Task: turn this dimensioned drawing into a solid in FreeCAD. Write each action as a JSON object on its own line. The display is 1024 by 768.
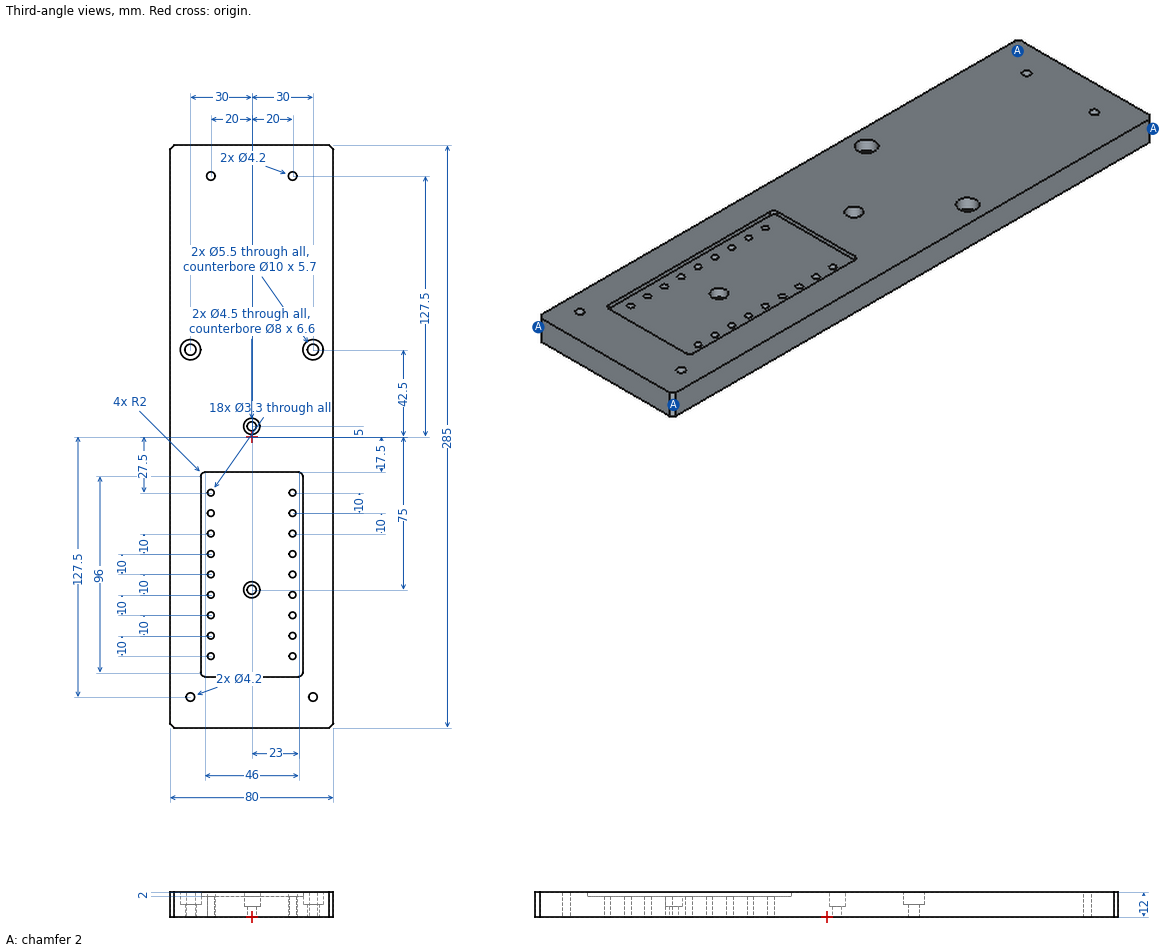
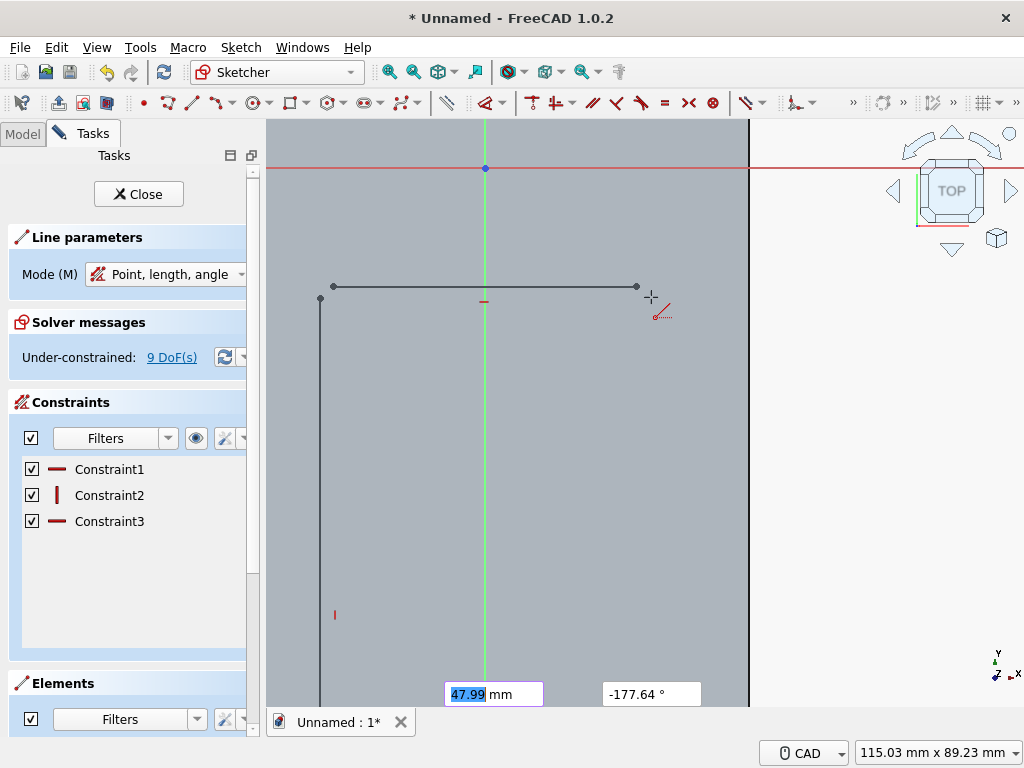
{"action": "left_click", "coordinate": [650, 297]}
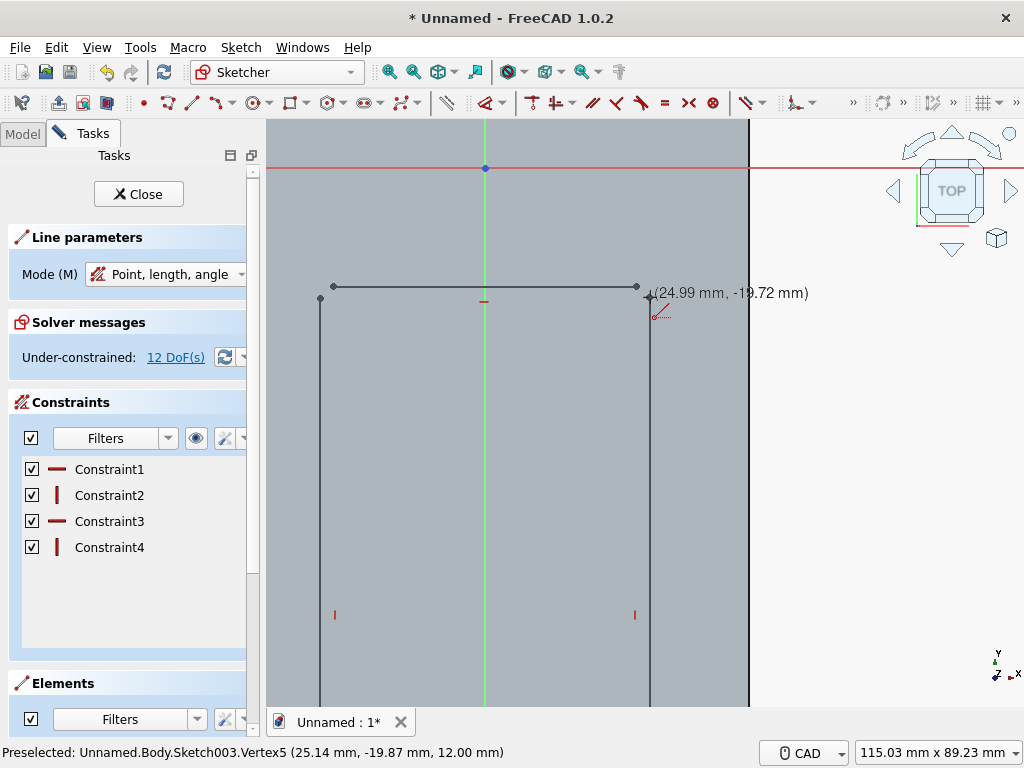
{"action": "key", "text": "g 3 a"}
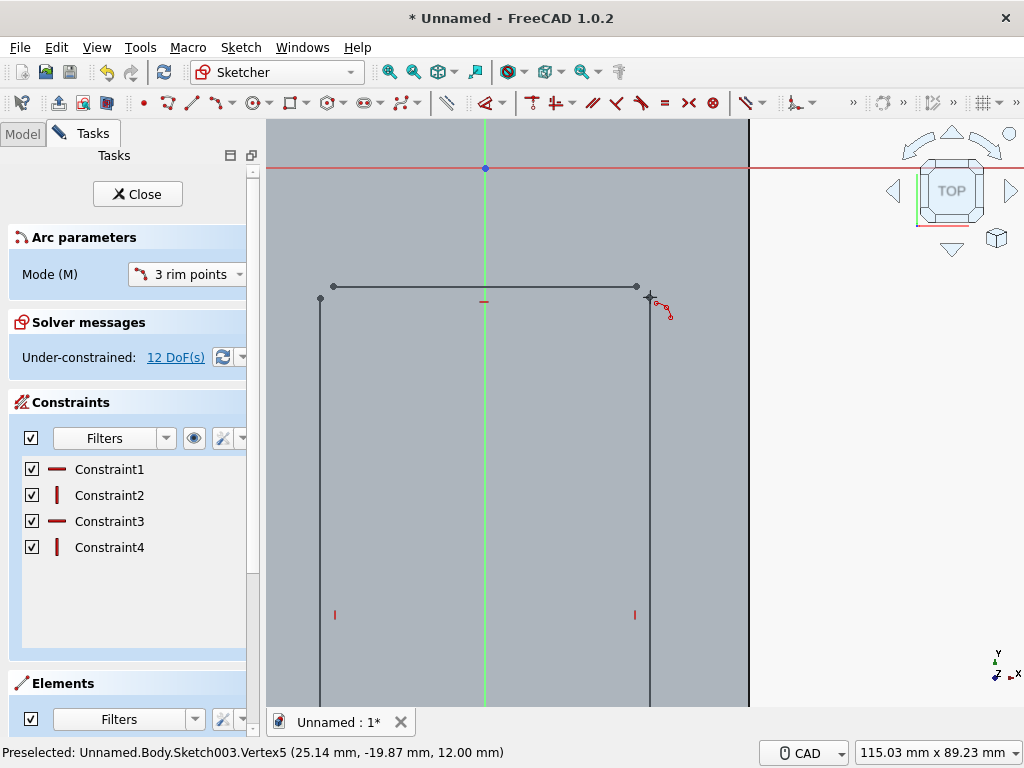
{"action": "left_click", "coordinate": [333, 287]}
{"action": "left_click", "coordinate": [320, 298]}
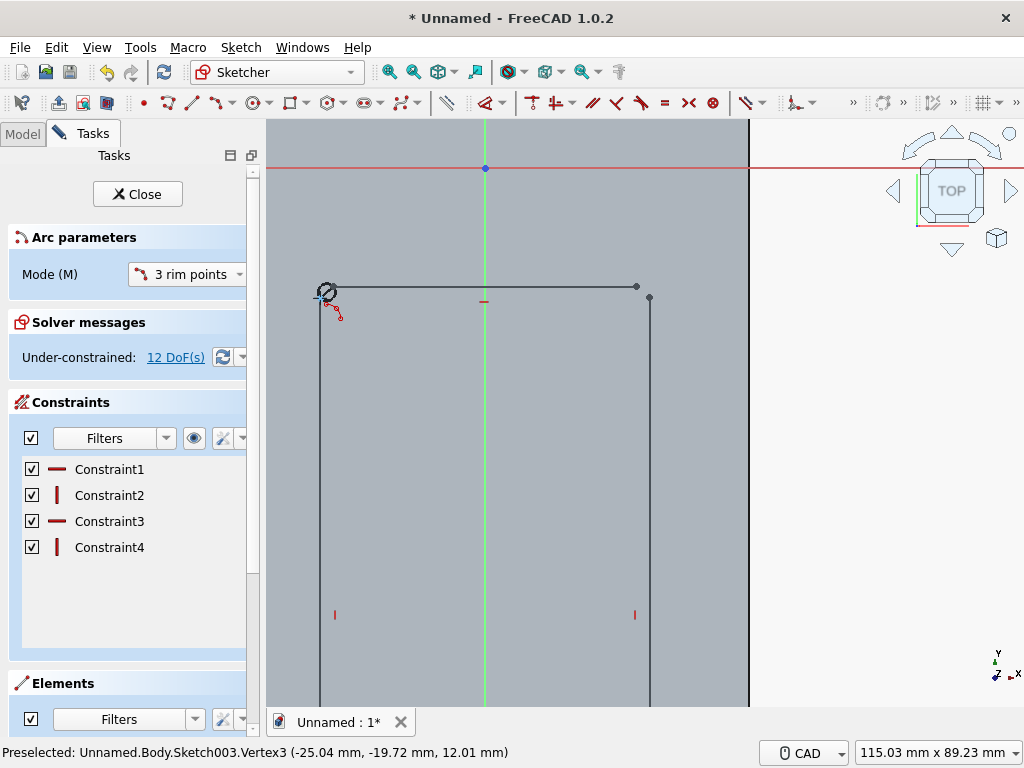
{"action": "scroll", "coordinate": [324, 287], "scroll_direction": "up", "scroll_amount": 8}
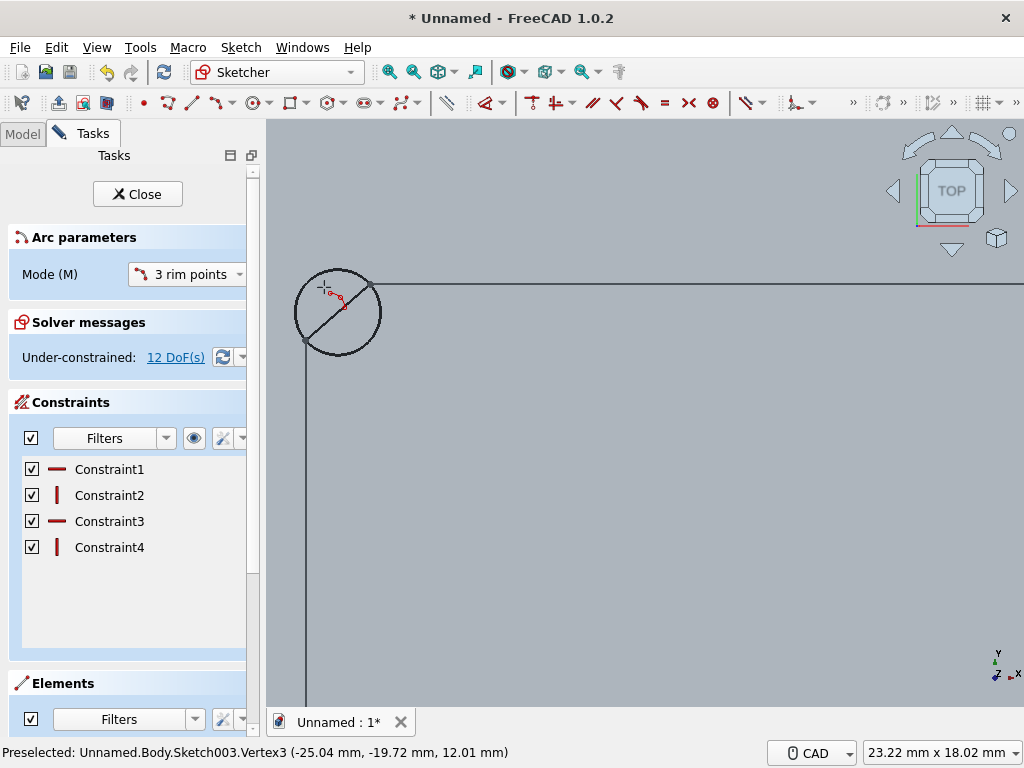
{"action": "left_click", "coordinate": [326, 287]}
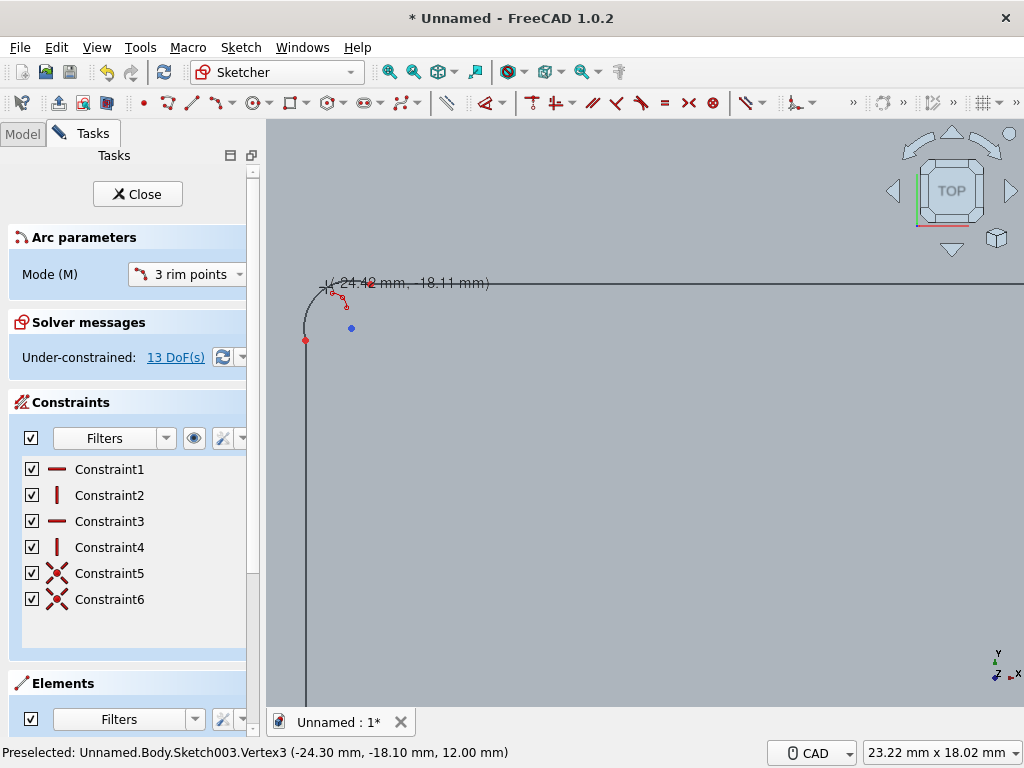
{"action": "scroll", "coordinate": [522, 293], "scroll_direction": "down", "scroll_amount": 12}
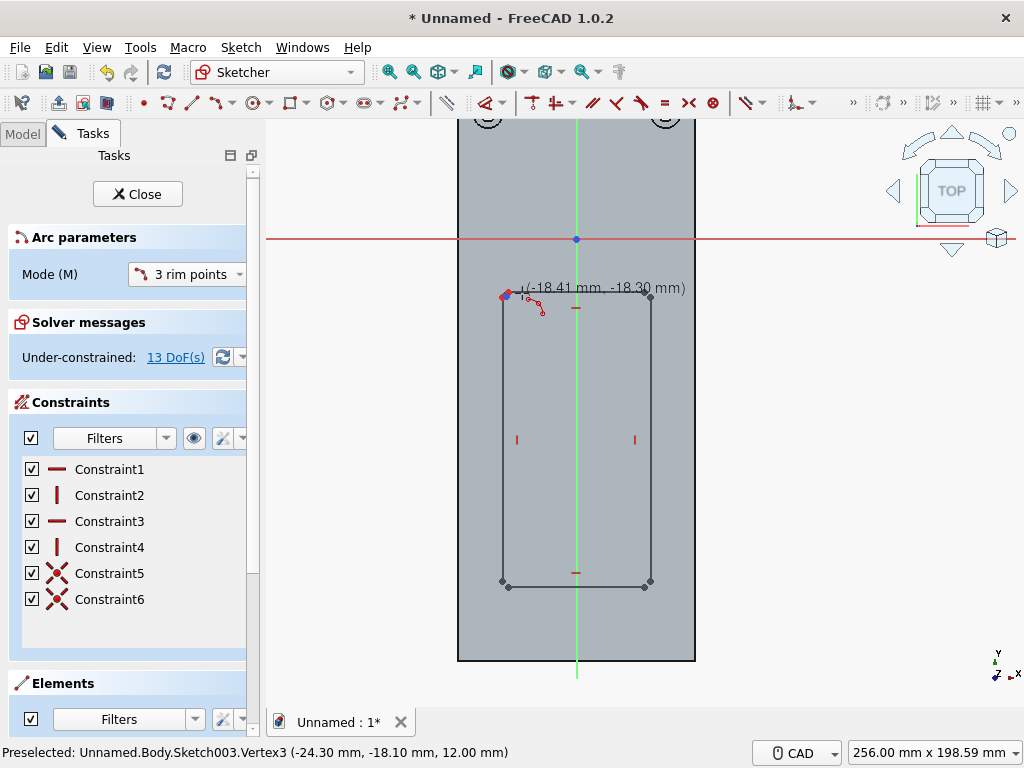
{"action": "scroll", "coordinate": [503, 581], "scroll_direction": "up", "scroll_amount": 4}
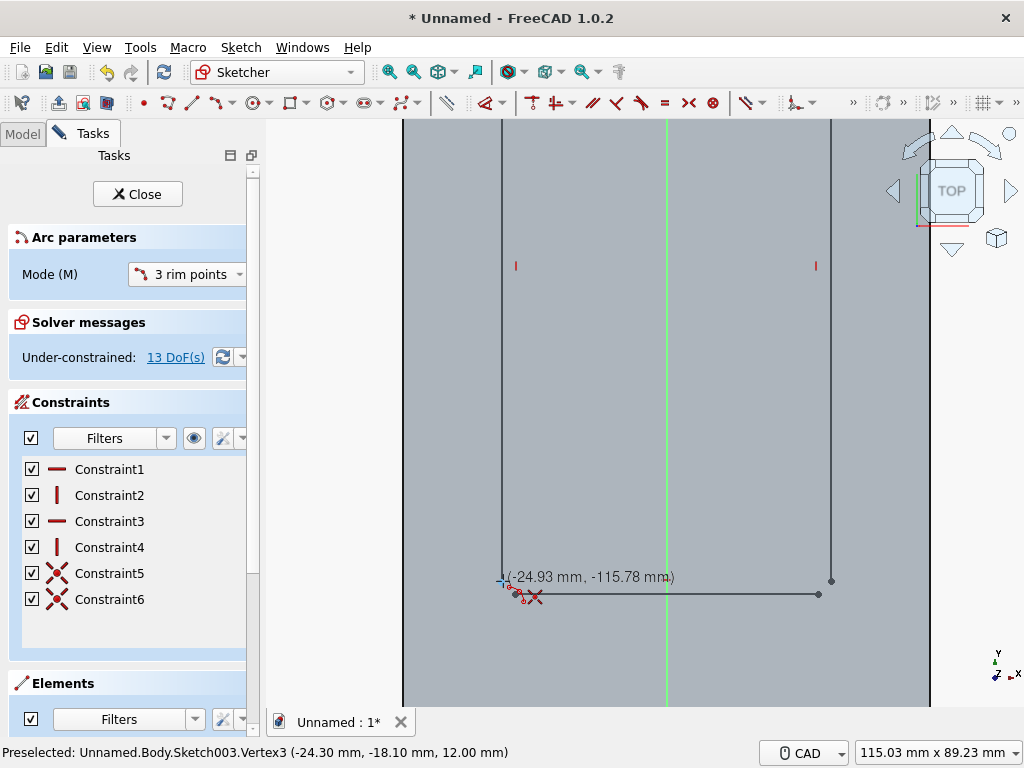
{"action": "left_click", "coordinate": [502, 582]}
{"action": "left_click", "coordinate": [515, 594]}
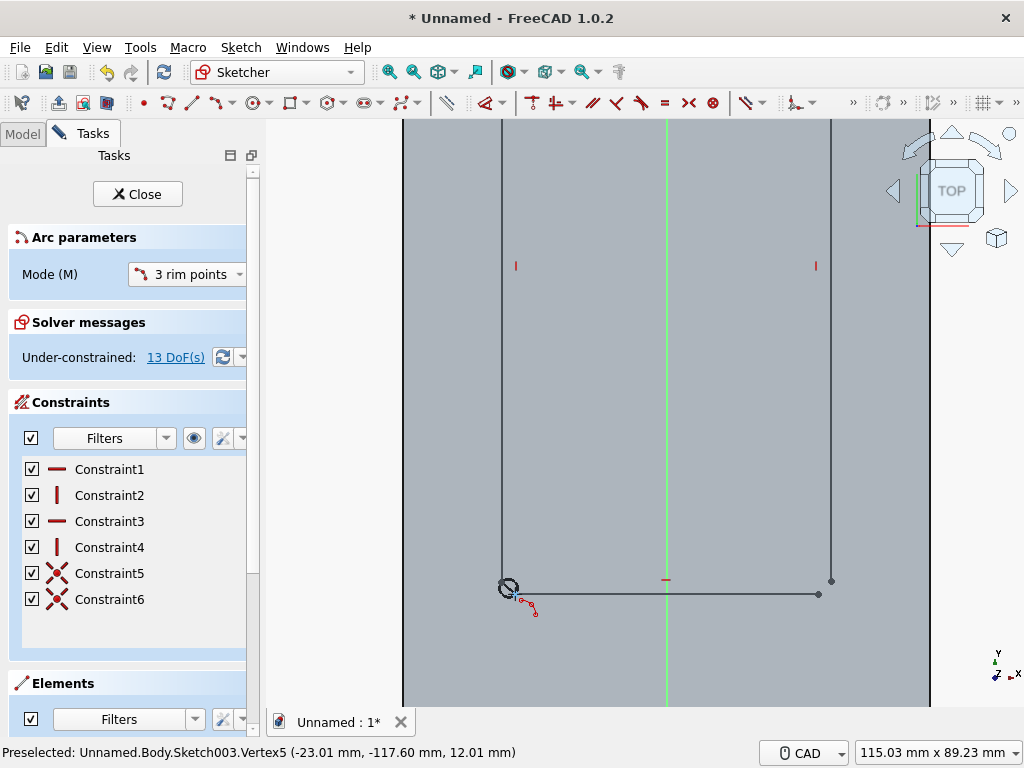
{"action": "scroll", "coordinate": [506, 590], "scroll_direction": "up", "scroll_amount": 8}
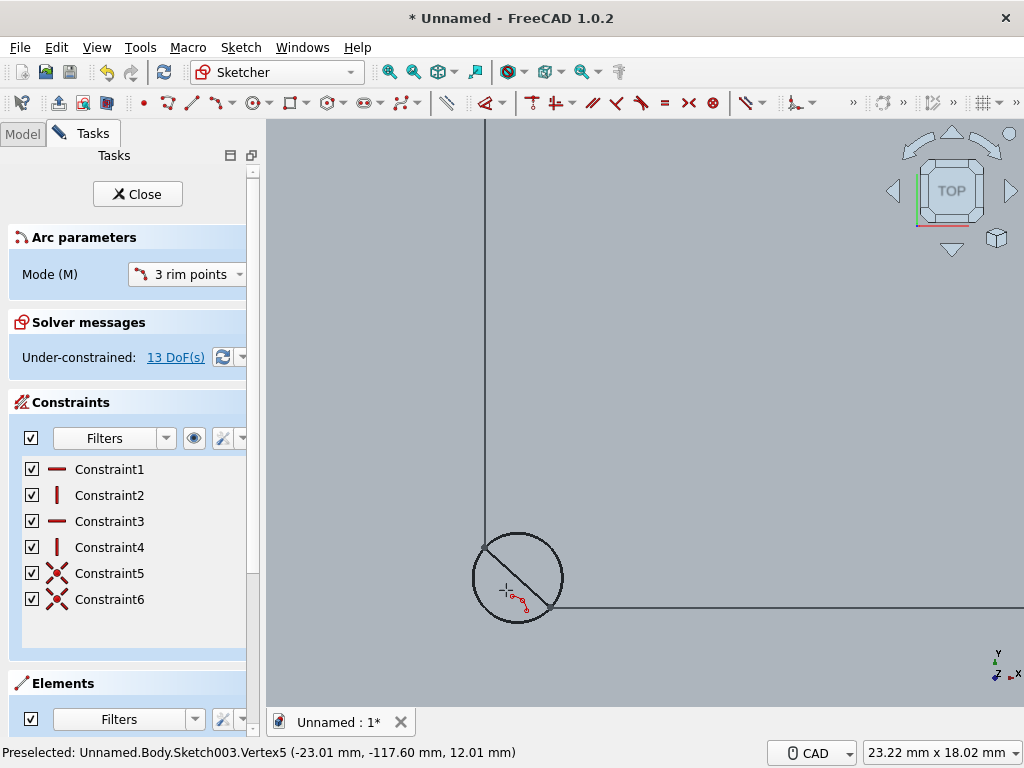
{"action": "left_click", "coordinate": [505, 585]}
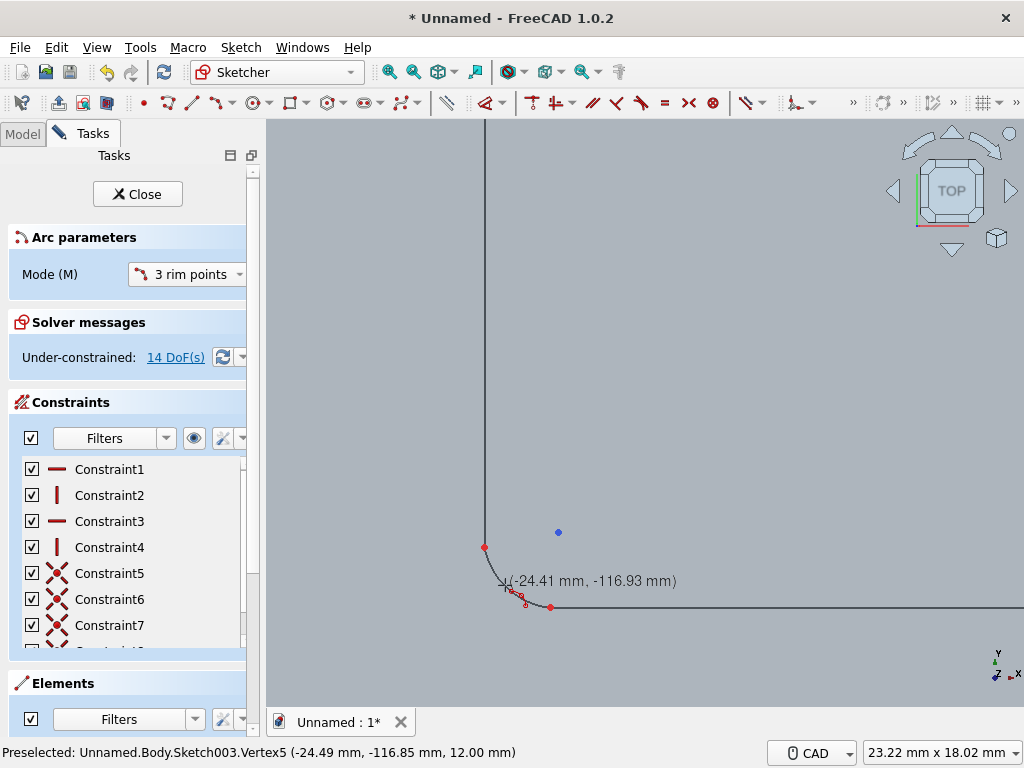
{"action": "scroll", "coordinate": [504, 585], "scroll_direction": "down", "scroll_amount": 12}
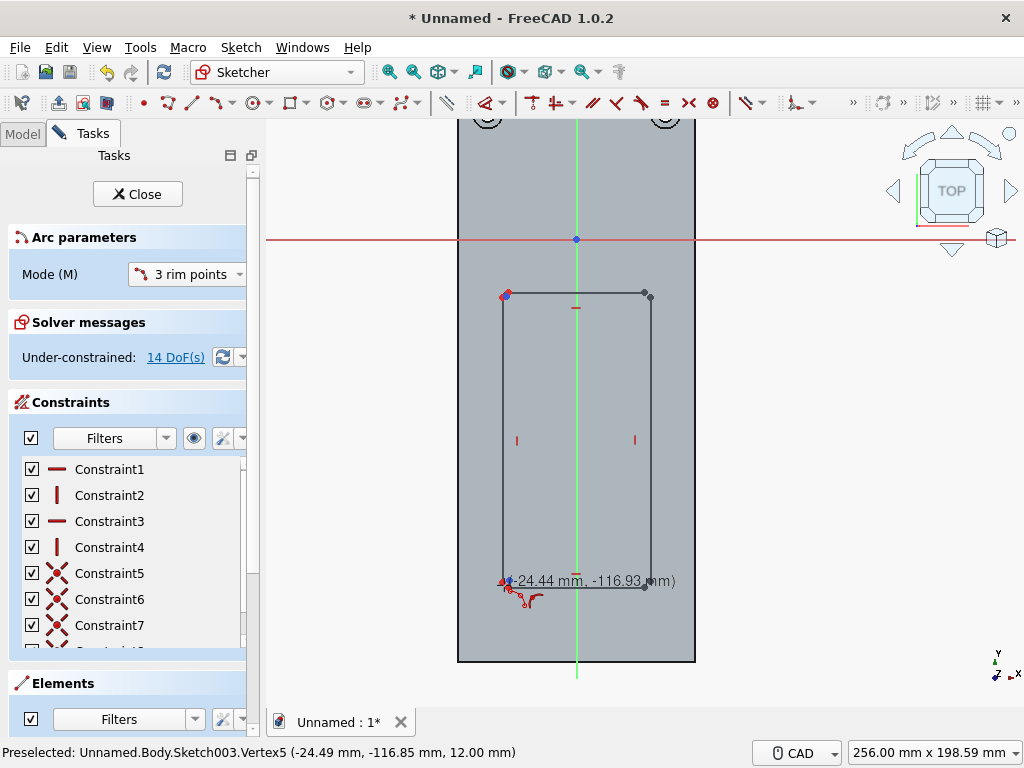
{"action": "scroll", "coordinate": [645, 587], "scroll_direction": "up", "scroll_amount": 4}